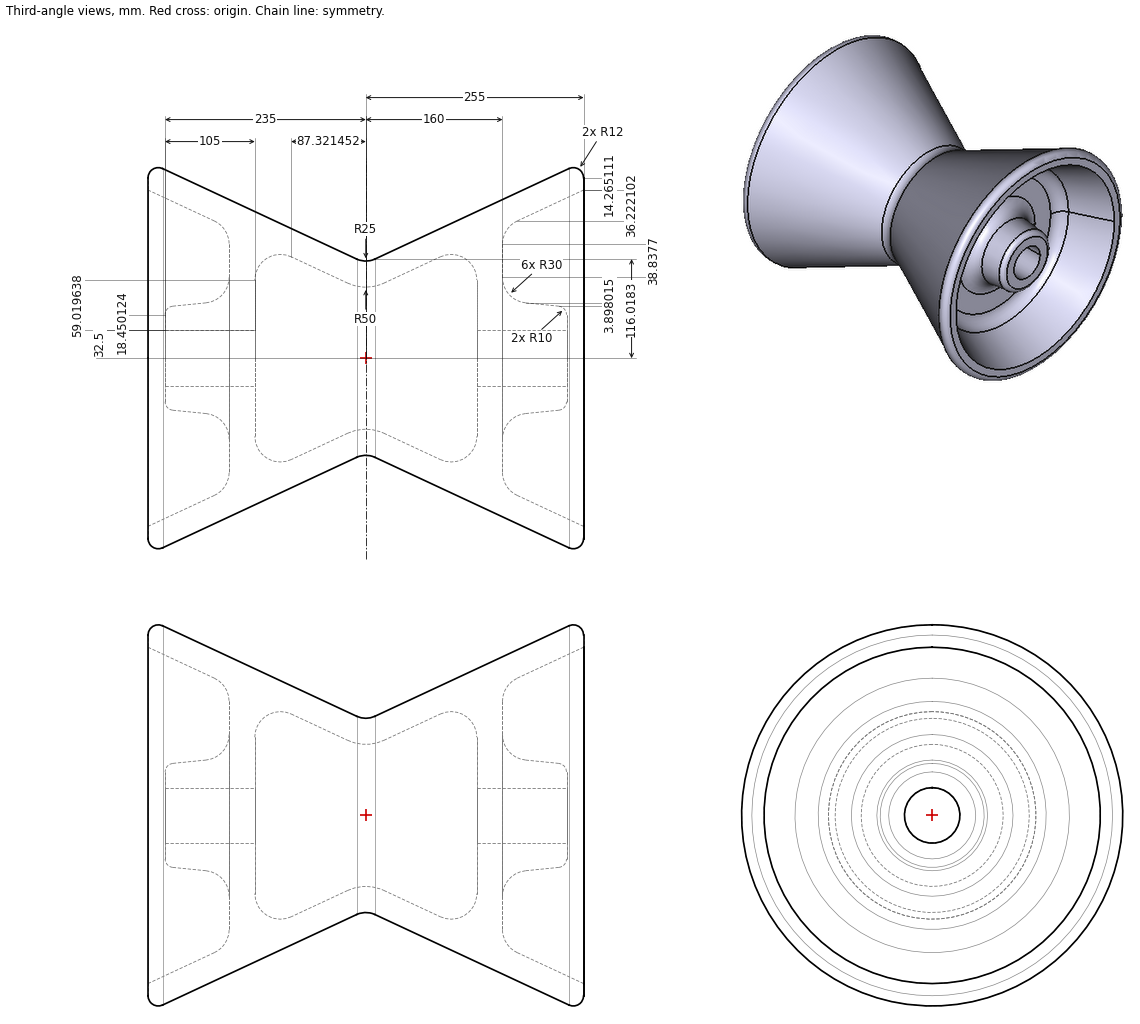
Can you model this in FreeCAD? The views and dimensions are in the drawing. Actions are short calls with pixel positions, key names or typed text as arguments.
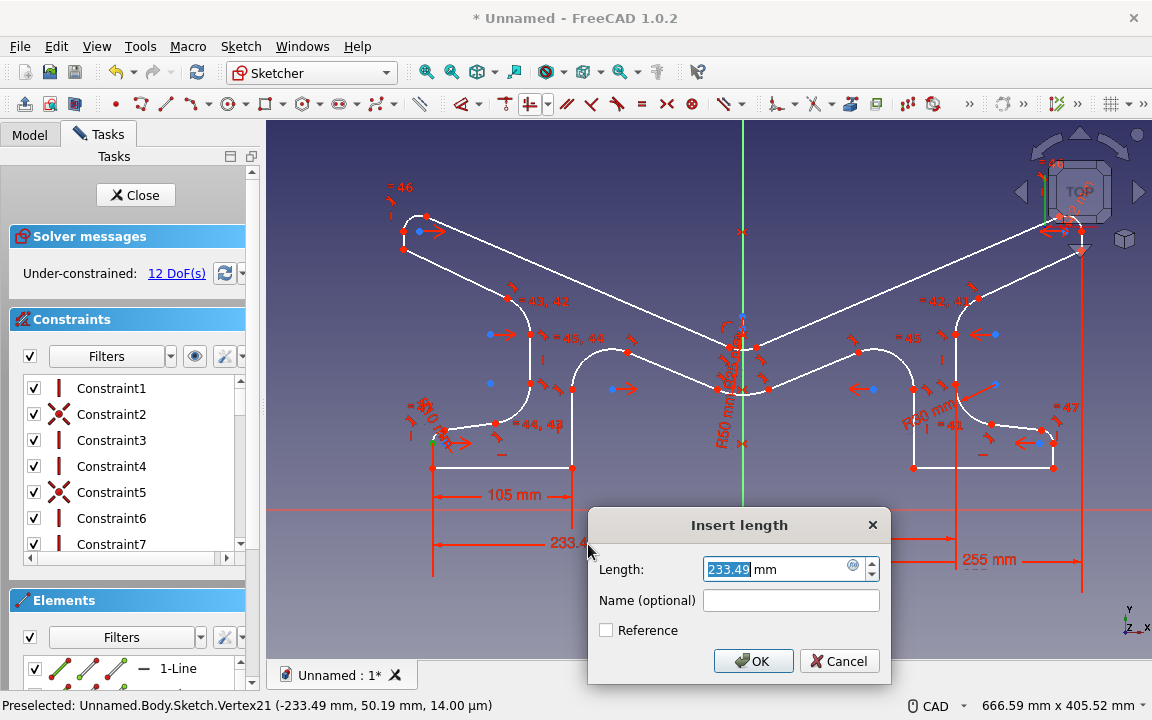
text(235)
key(Return)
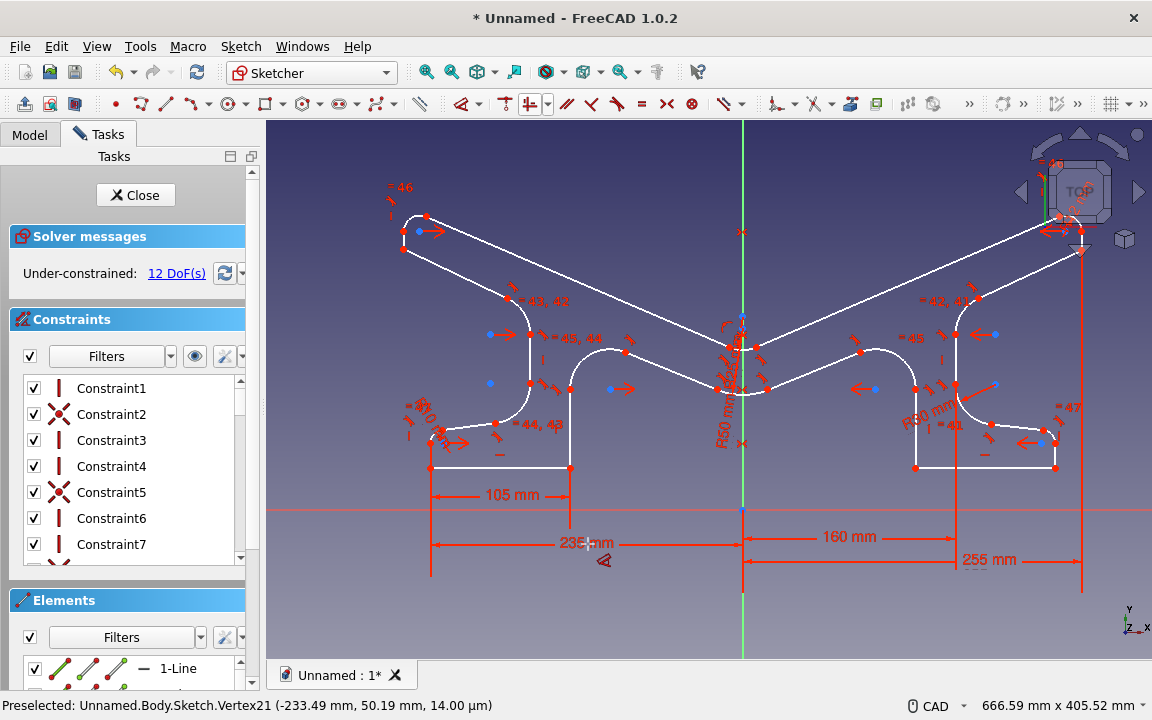
click(431, 468)
click(397, 489)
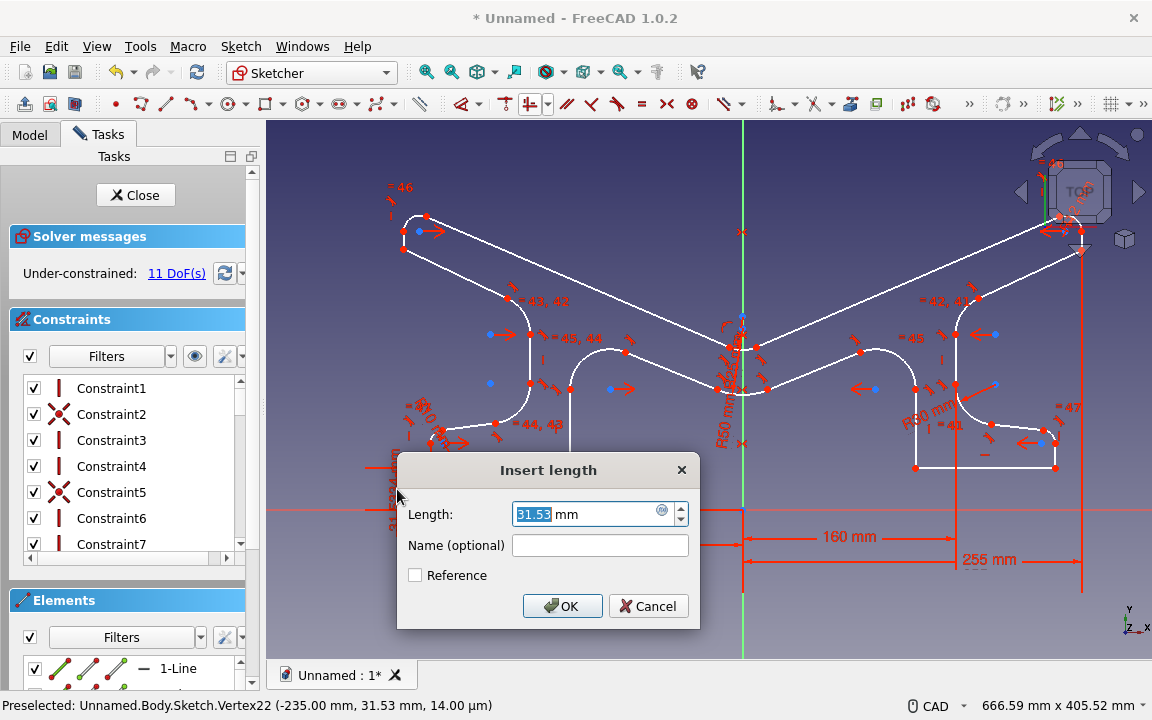
text(32.5)
key(Return)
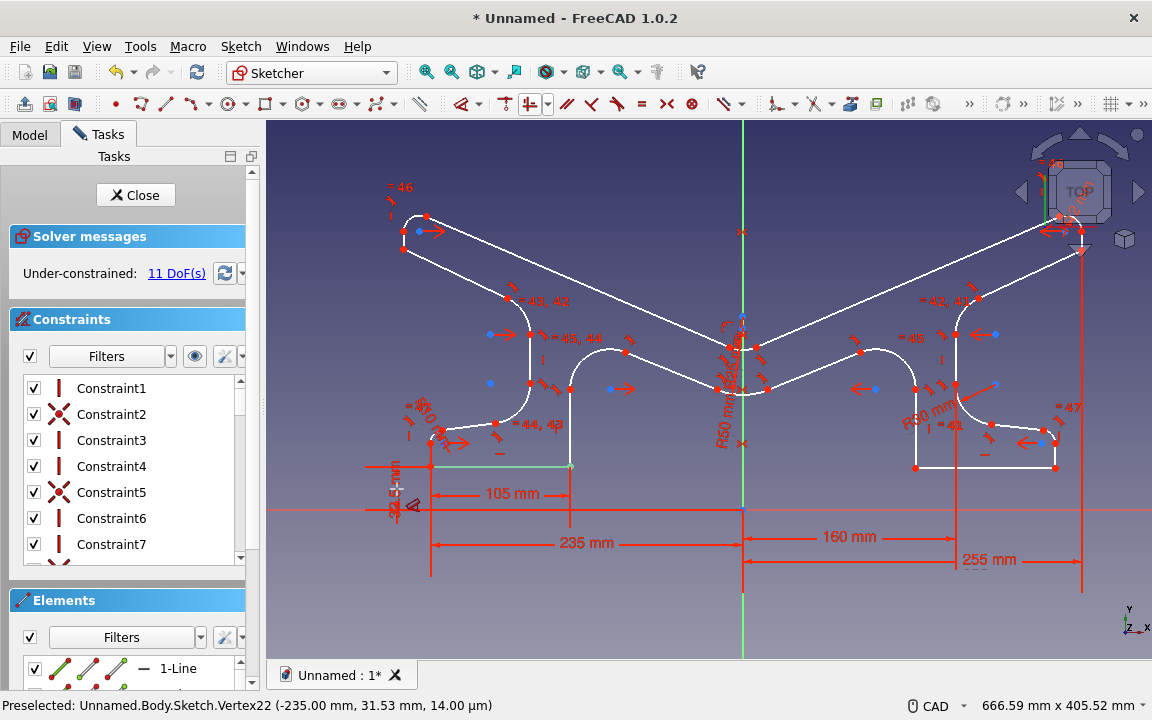
click(916, 468)
click(950, 489)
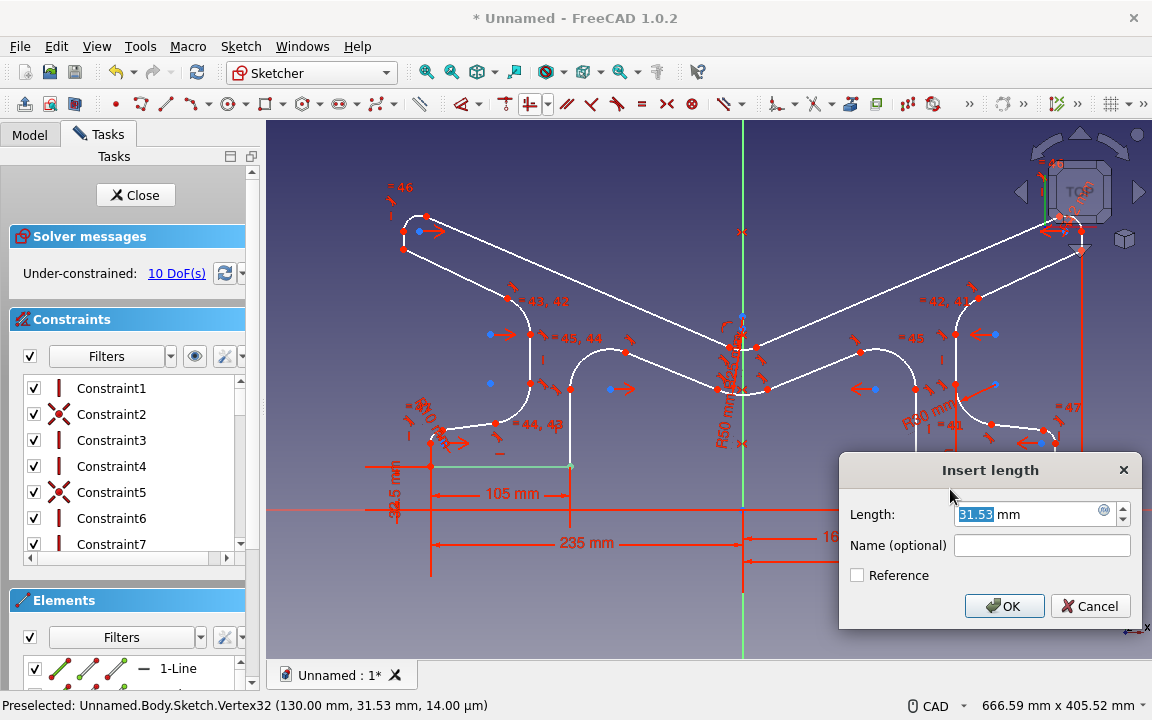
text(32.5)
key(Return)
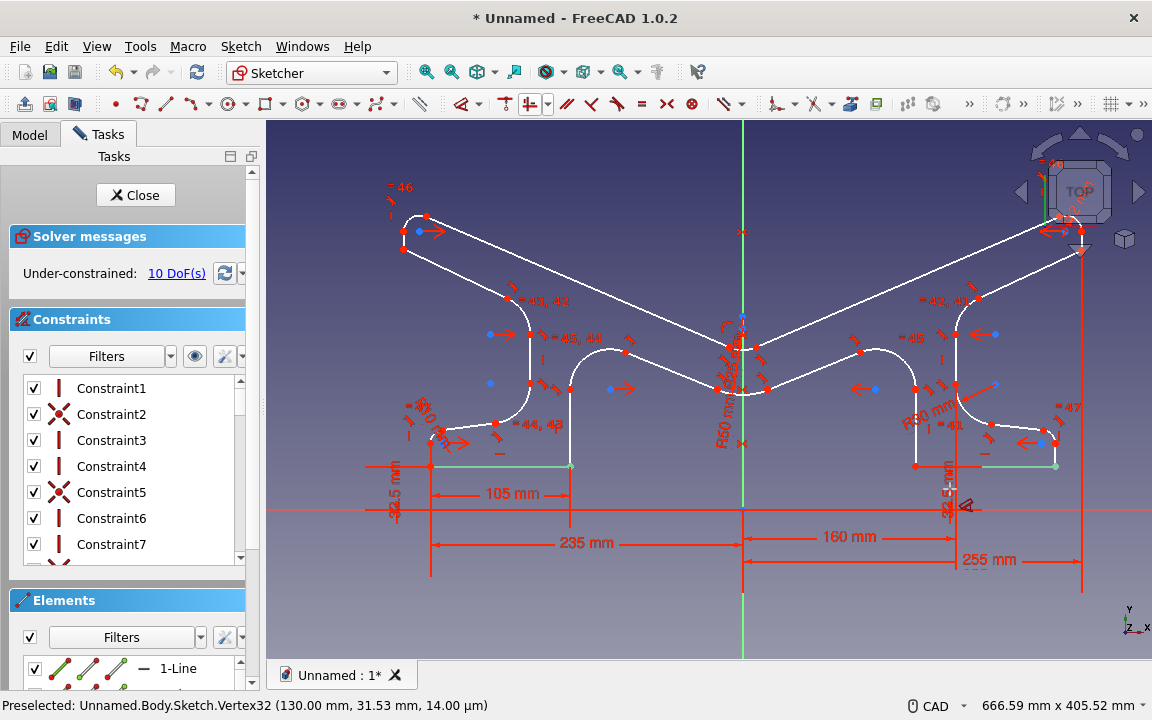
click(956, 370)
click(922, 360)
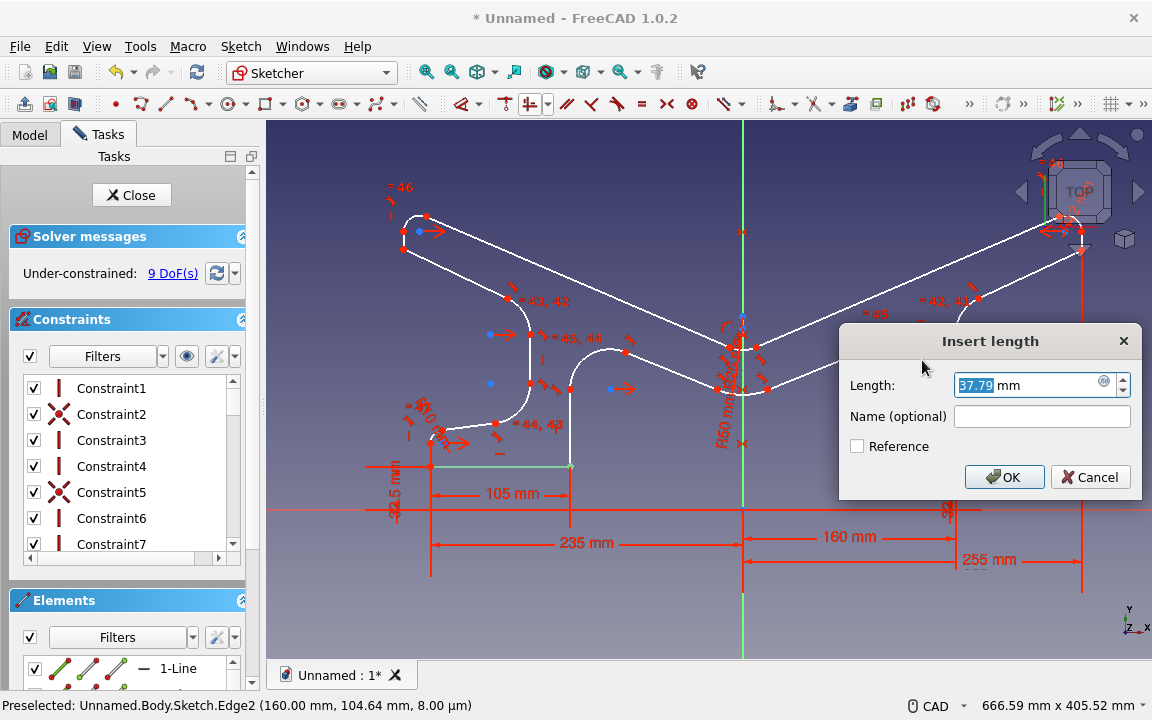
text(38.8377)
key(Return)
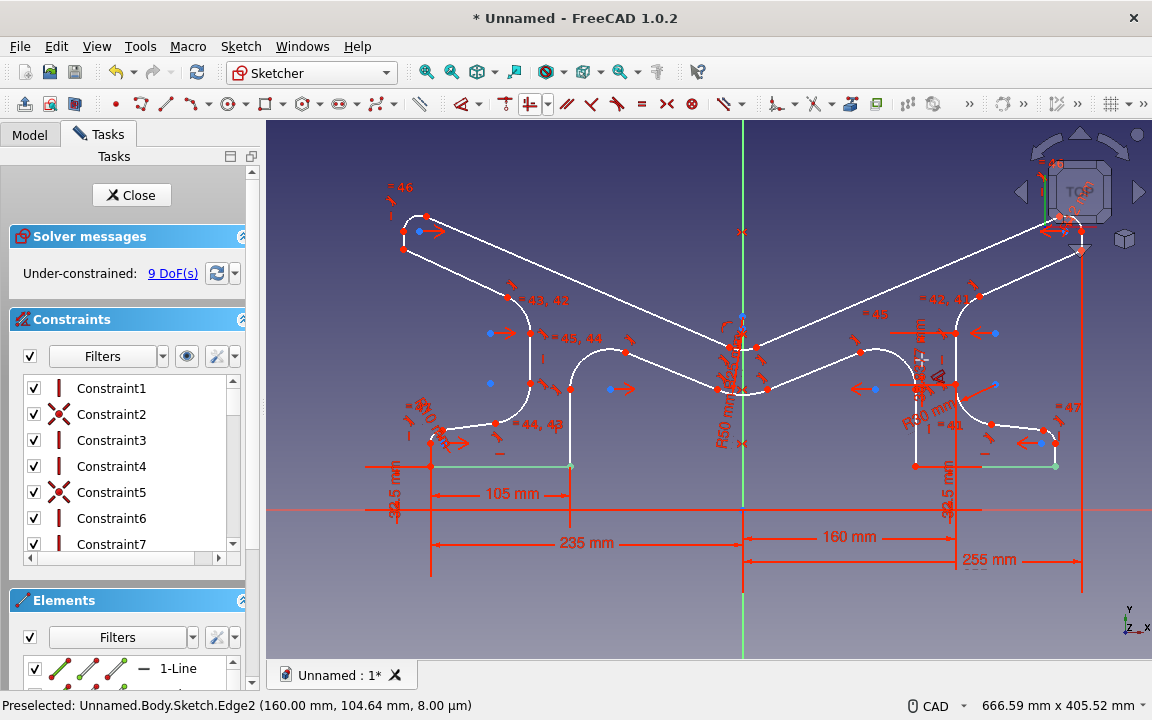
click(530, 348)
click(496, 358)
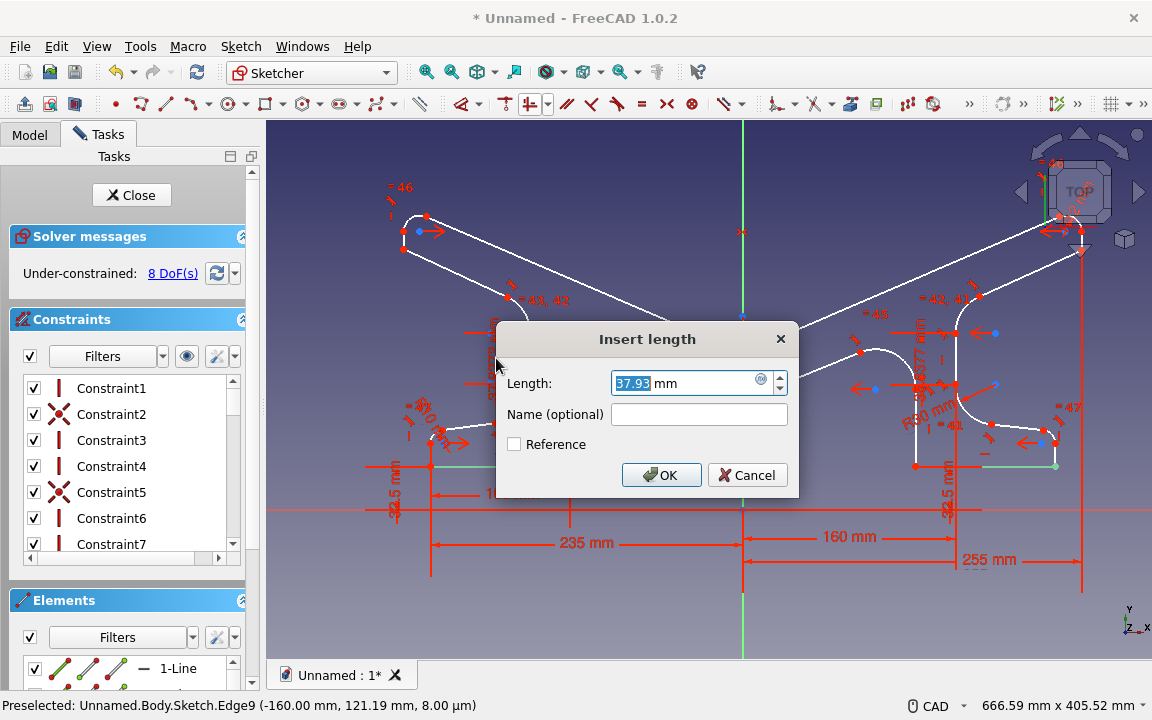
text(38.8377)
key(Return)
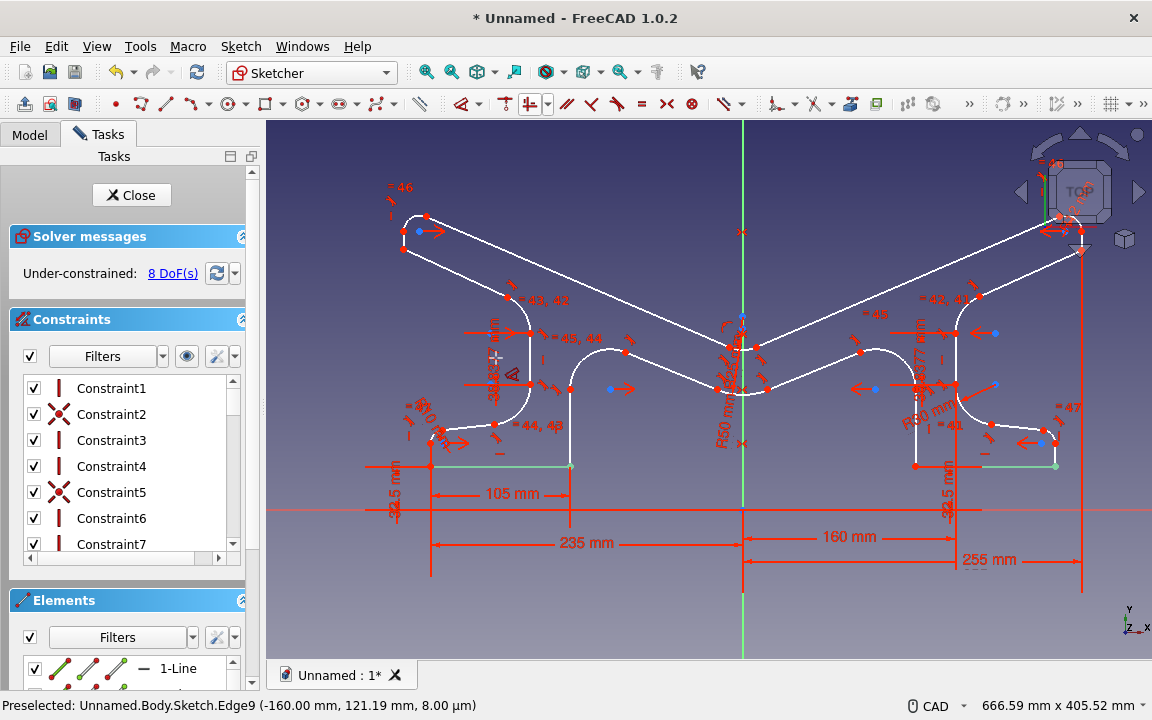
scroll(432, 444, down, 2)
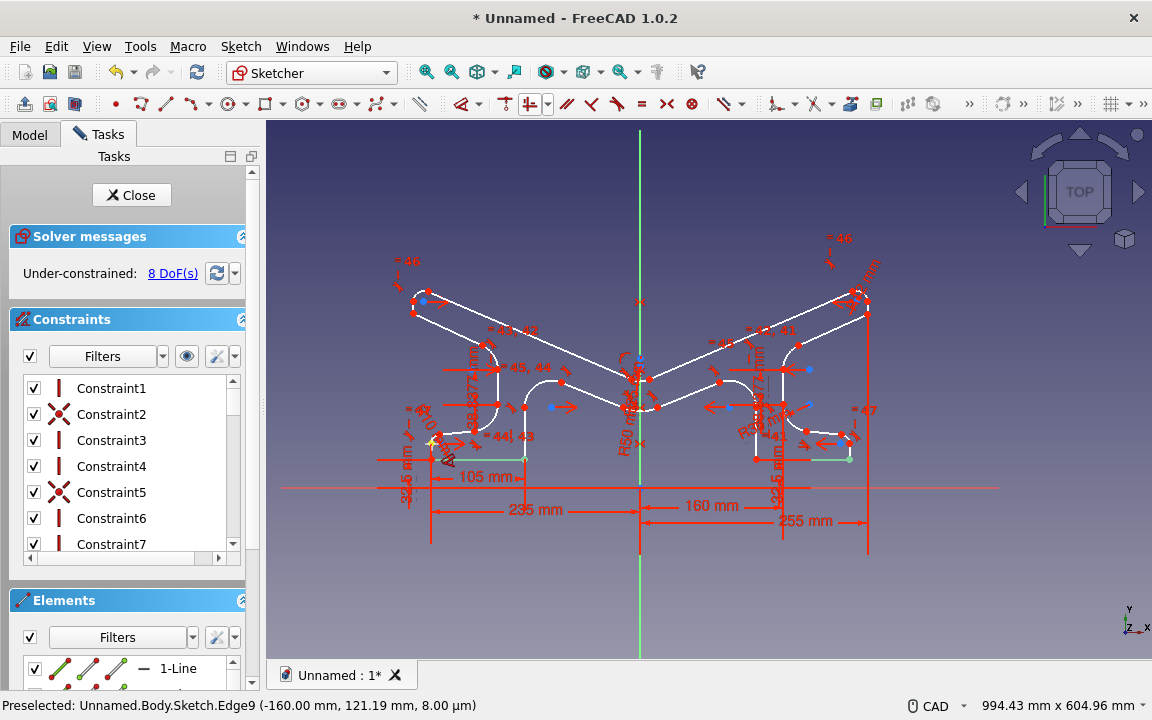
scroll(868, 308, up, 6)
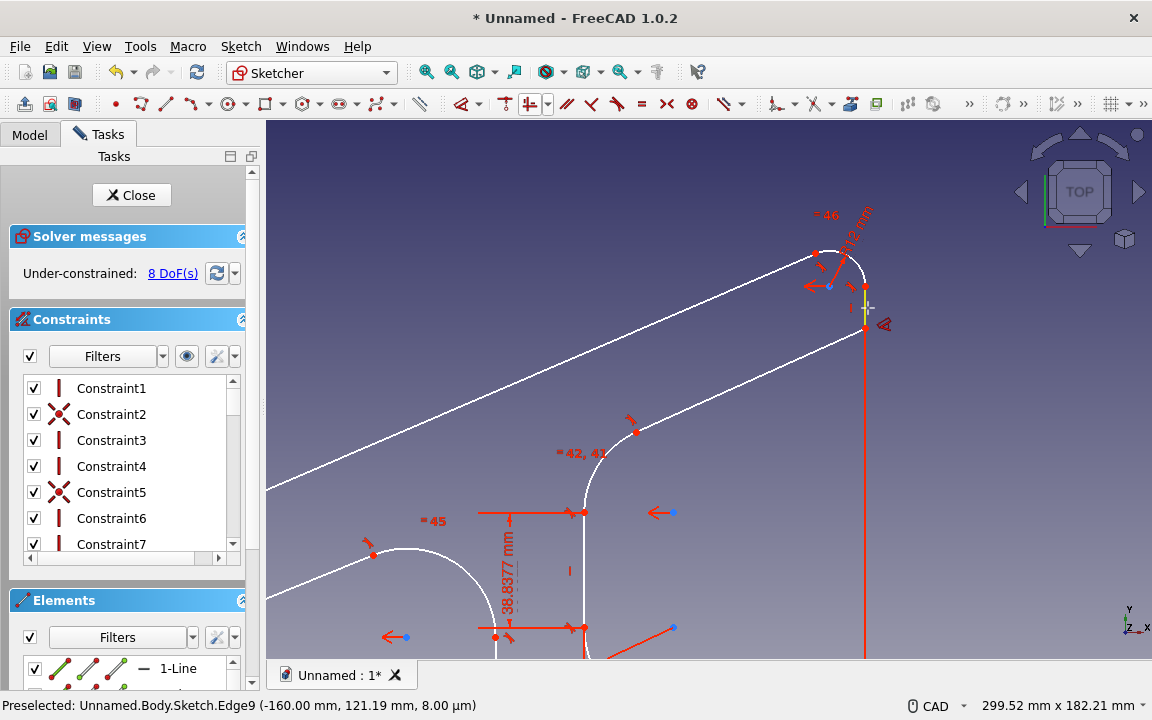
click(865, 308)
click(899, 308)